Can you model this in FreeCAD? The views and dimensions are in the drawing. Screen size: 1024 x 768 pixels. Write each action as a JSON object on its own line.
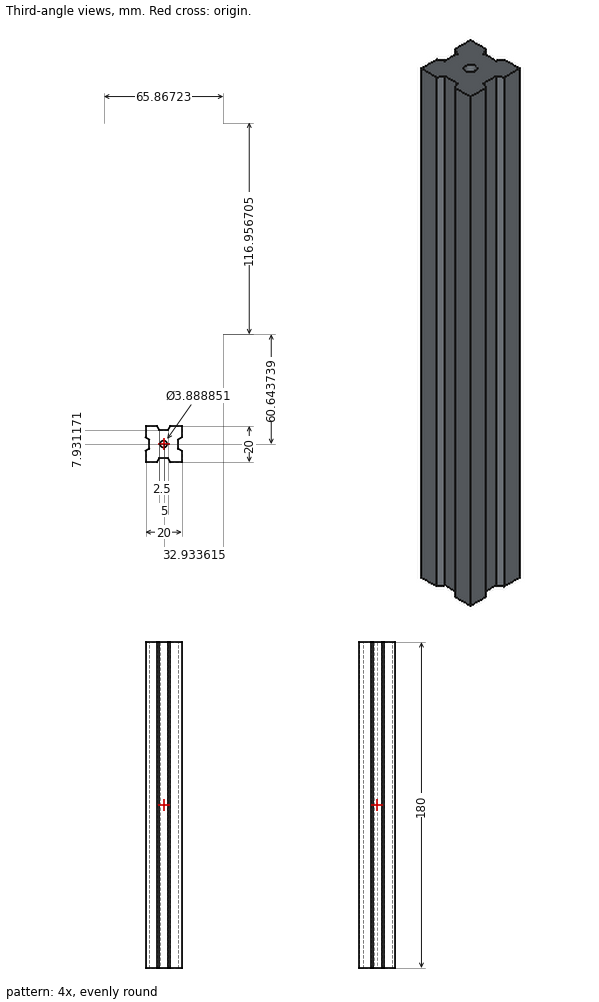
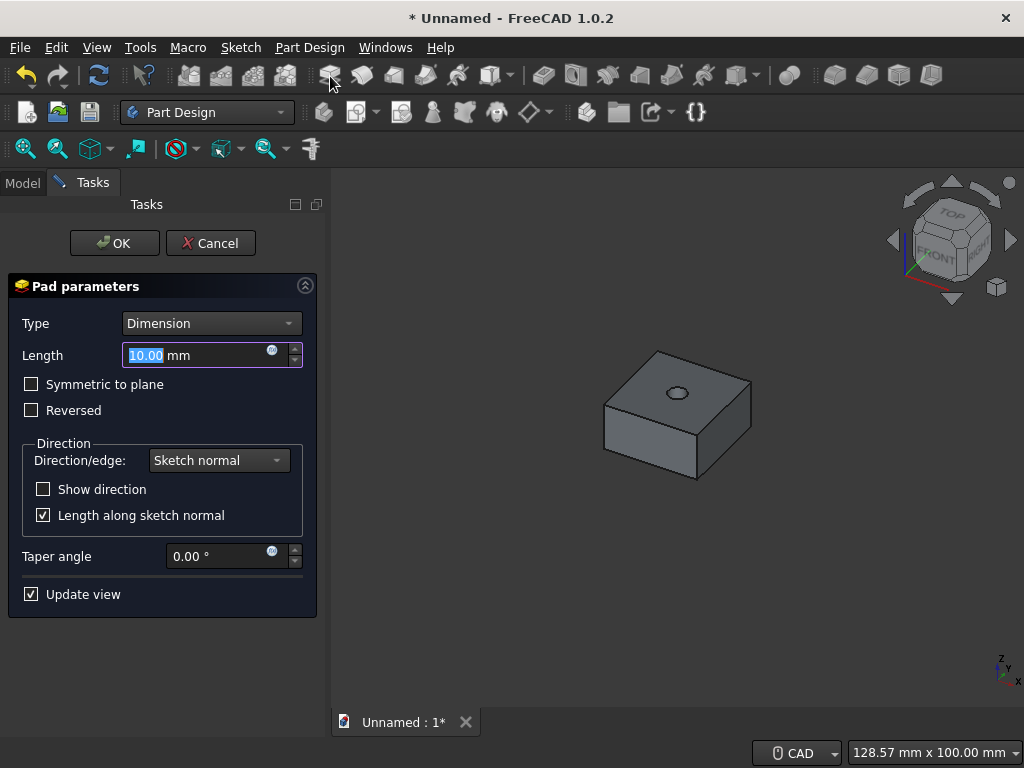
{"action": "type", "text": "180"}
{"action": "key", "text": "Tab"}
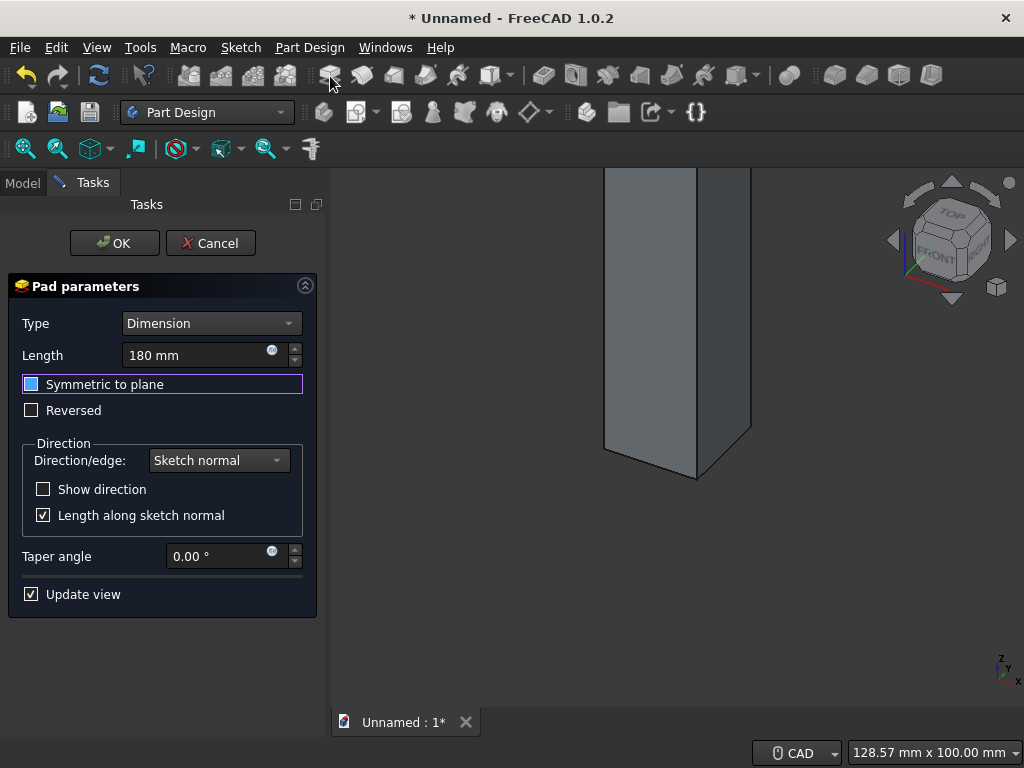
{"action": "left_click", "coordinate": [30, 384]}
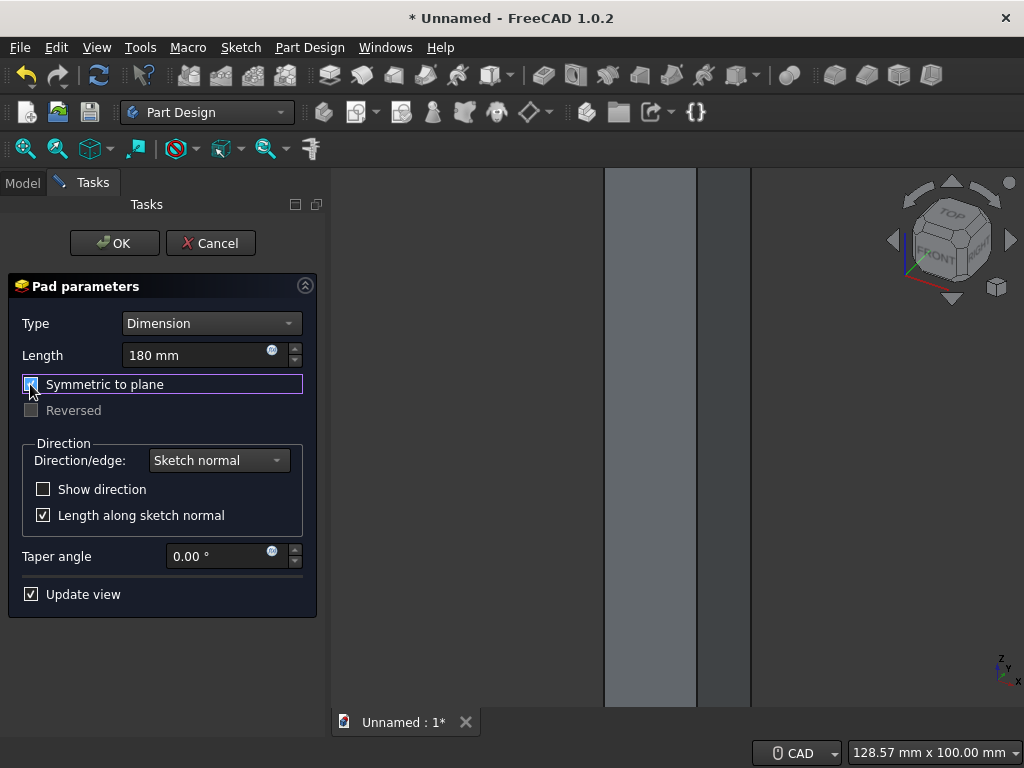
{"action": "left_click", "coordinate": [115, 243]}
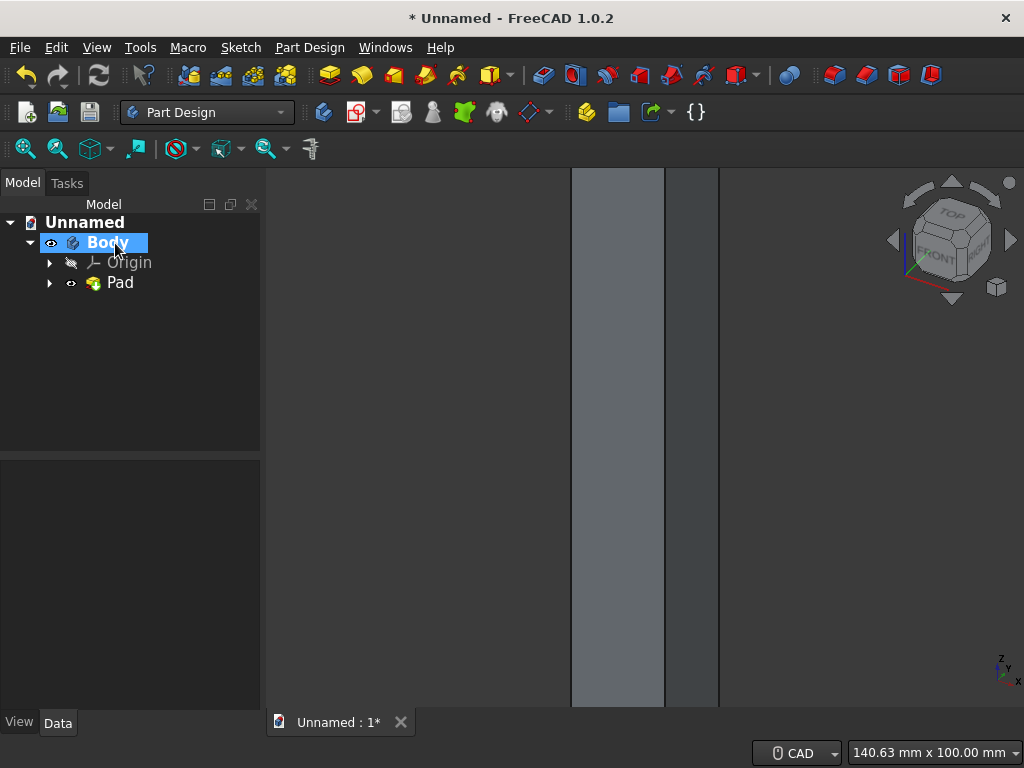
{"action": "left_click", "coordinate": [26, 150]}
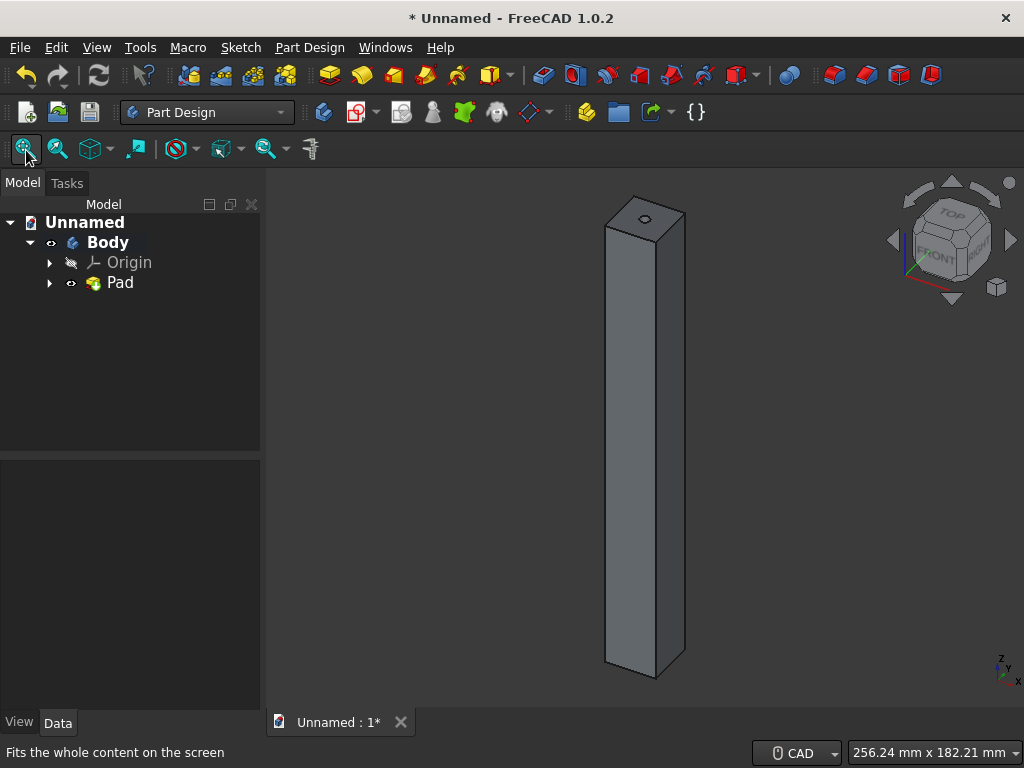
{"action": "left_click", "coordinate": [668, 215]}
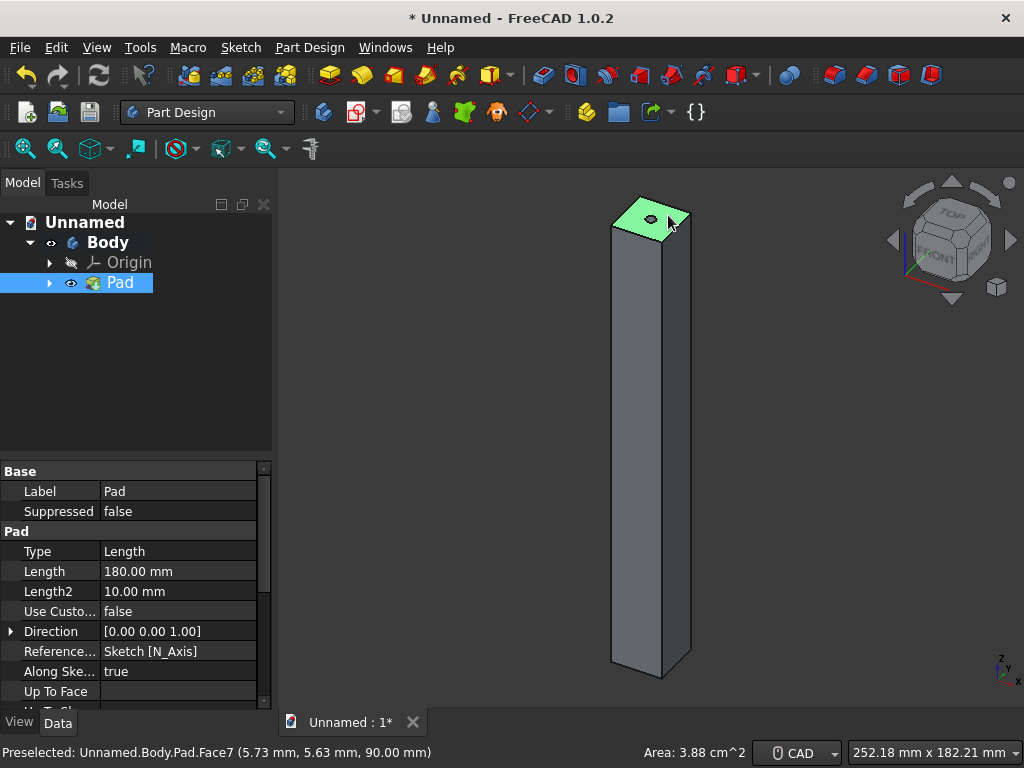
{"action": "left_click", "coordinate": [356, 112]}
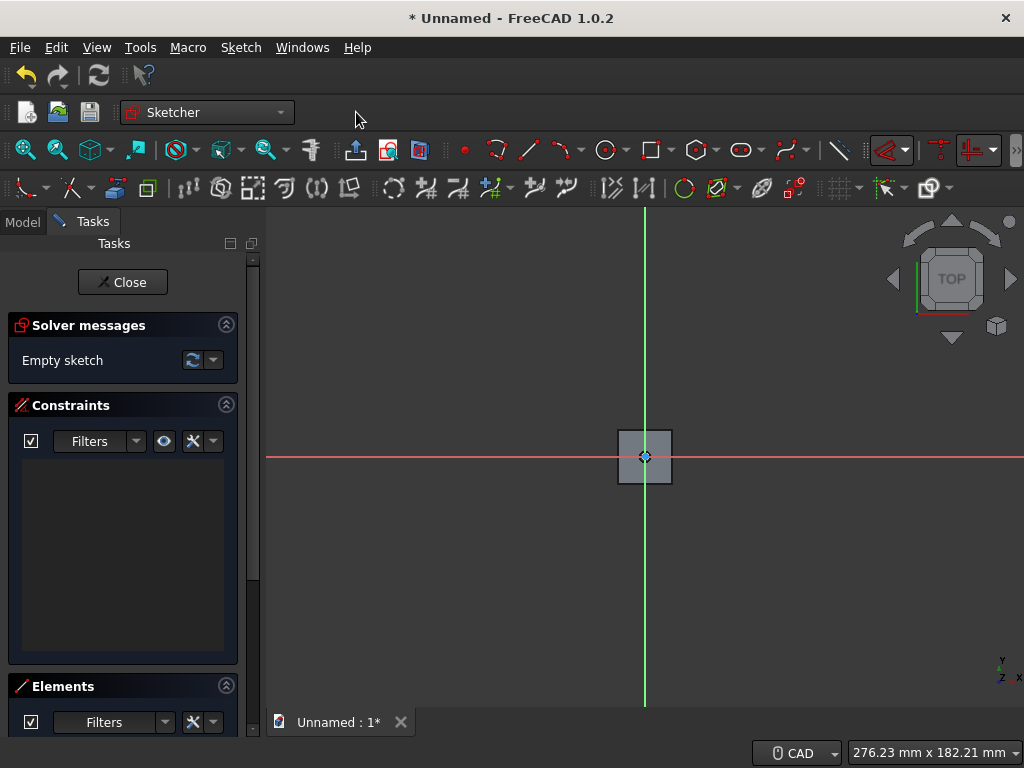
{"action": "scroll", "coordinate": [493, 679], "scroll_direction": "down", "scroll_amount": 3}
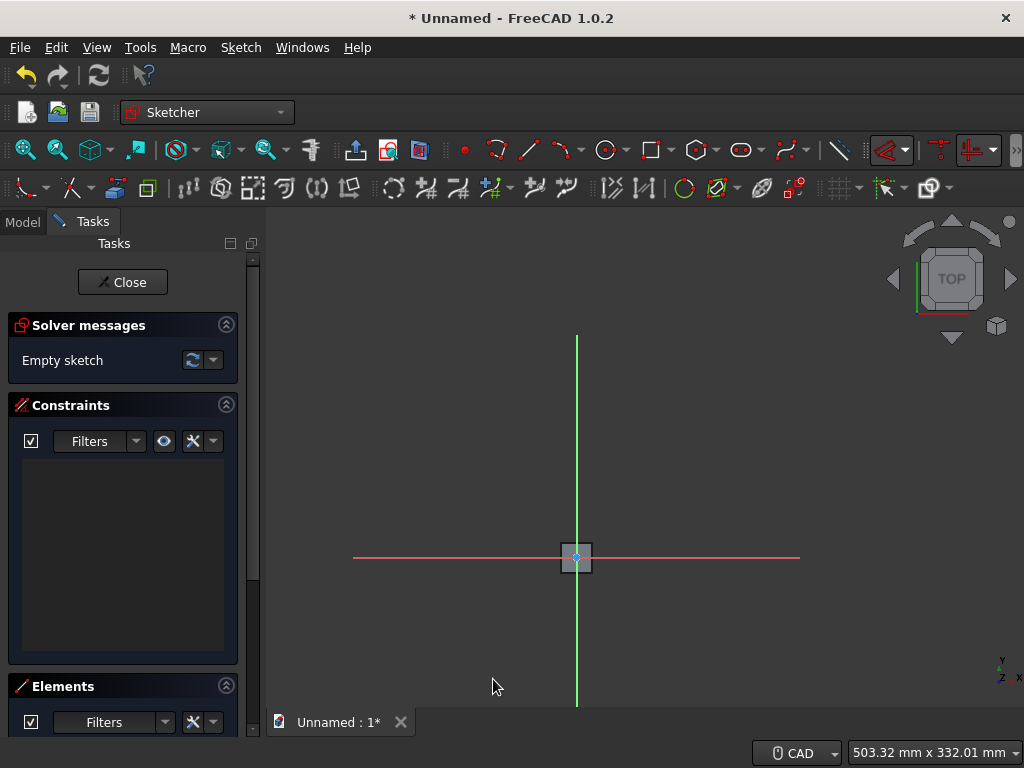
{"action": "left_click", "coordinate": [498, 150]}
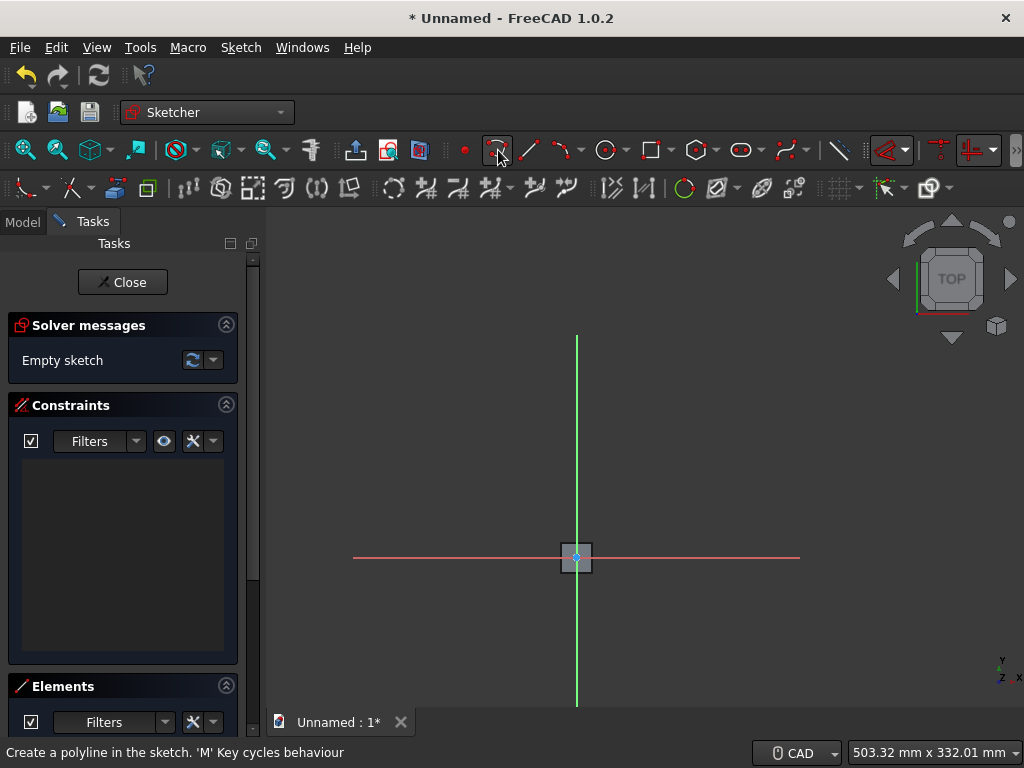
{"action": "scroll", "coordinate": [573, 546], "scroll_direction": "up", "scroll_amount": 8}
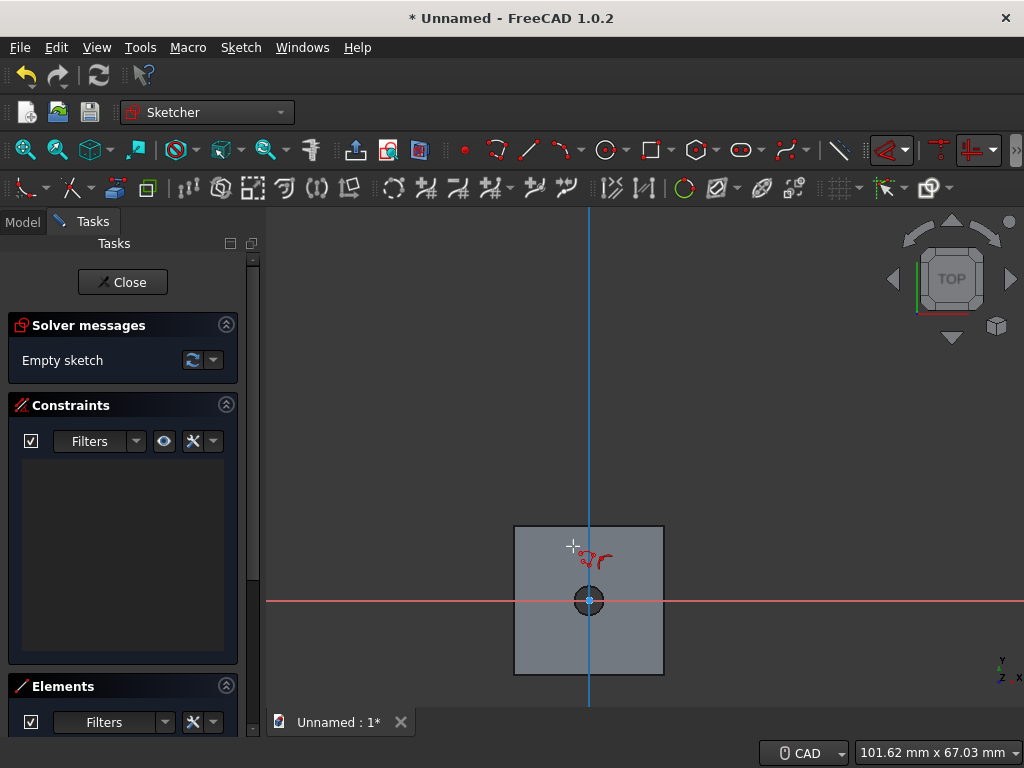
{"action": "left_click", "coordinate": [570, 542]}
{"action": "left_click", "coordinate": [608, 542]}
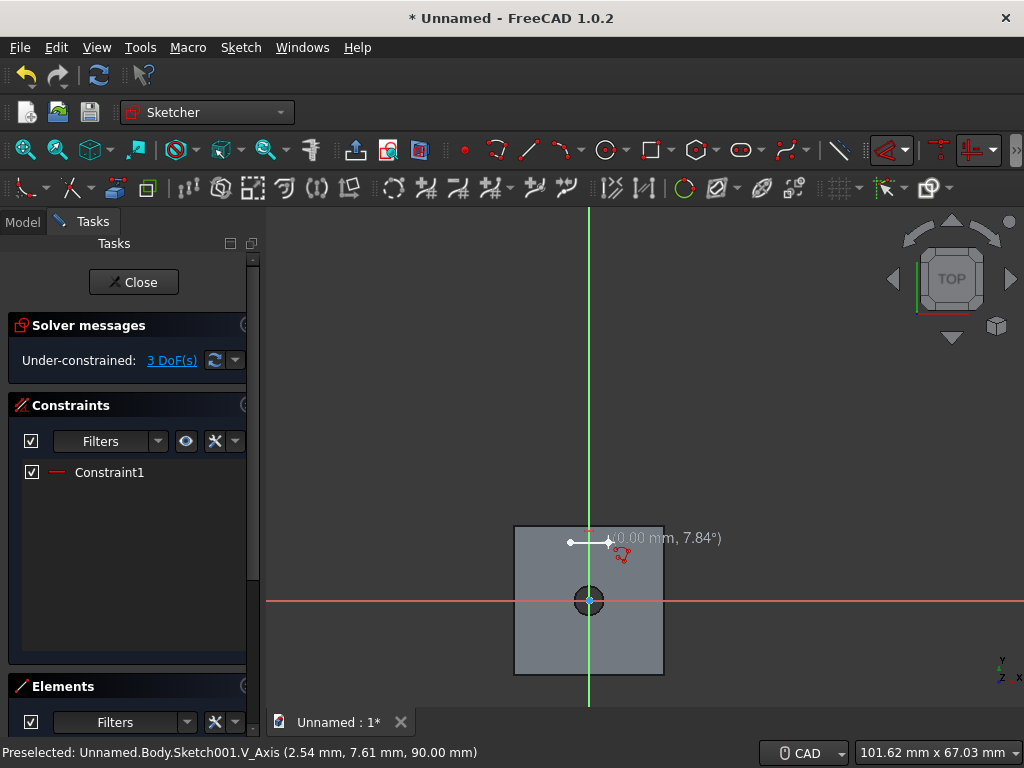
{"action": "scroll", "coordinate": [572, 627], "scroll_direction": "down", "scroll_amount": 7}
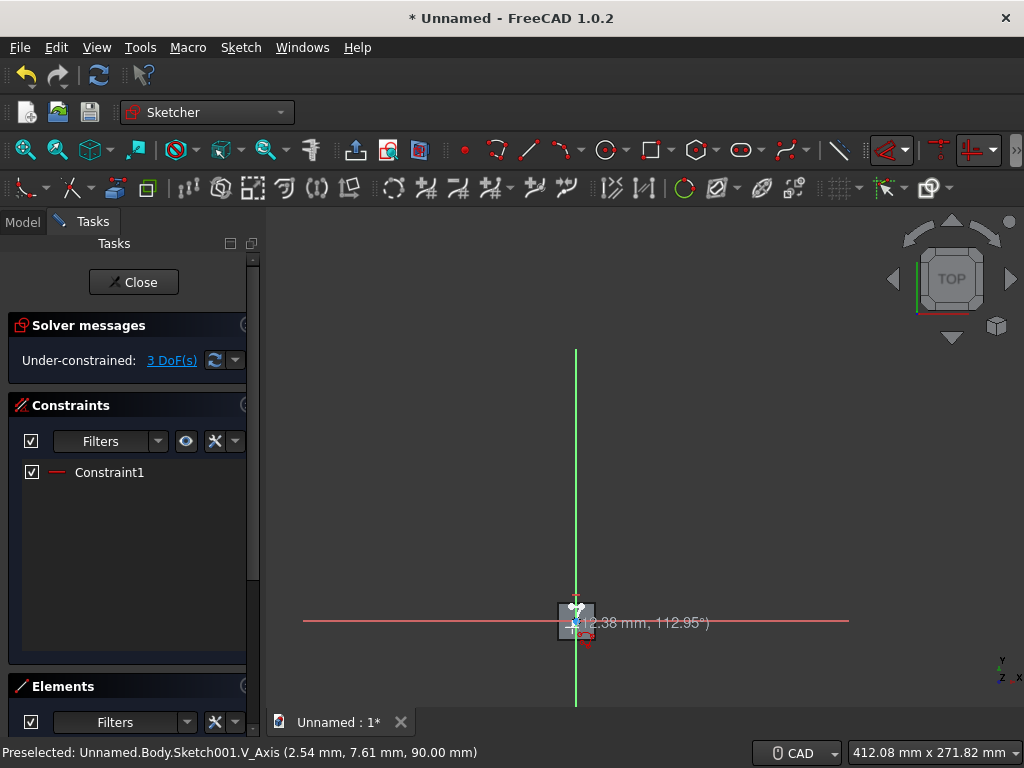
{"action": "left_click", "coordinate": [637, 510]}
{"action": "left_click", "coordinate": [637, 294]}
{"action": "left_click", "coordinate": [516, 294]}
{"action": "left_click", "coordinate": [516, 510]}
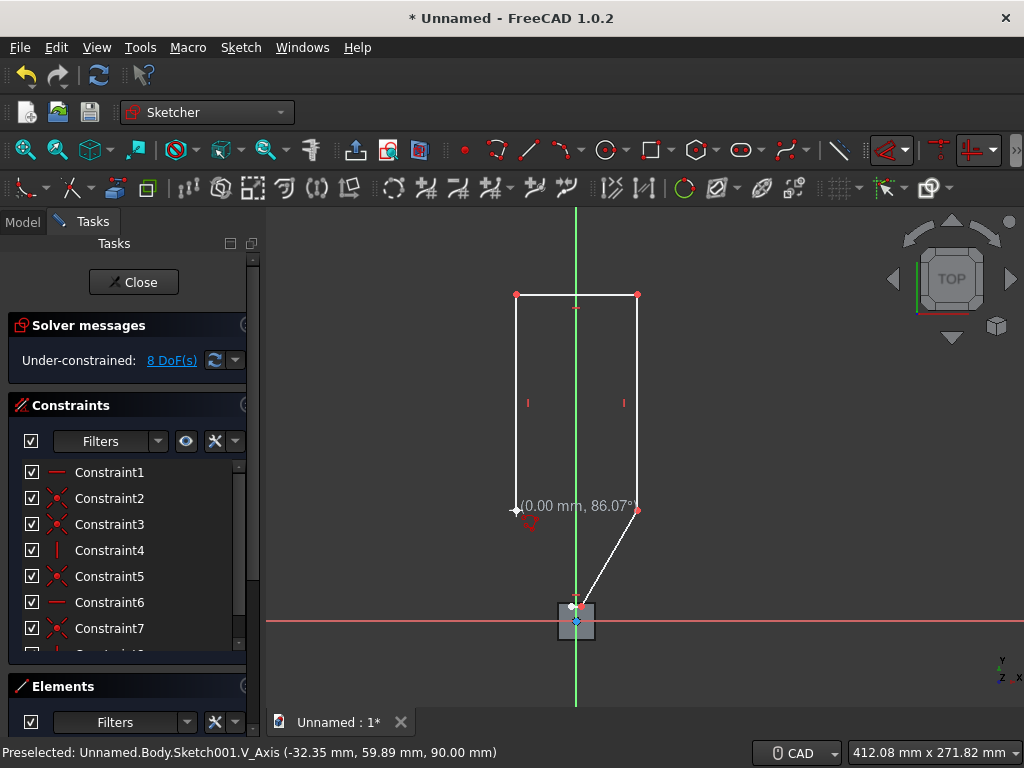
{"action": "scroll", "coordinate": [572, 607], "scroll_direction": "up", "scroll_amount": 7}